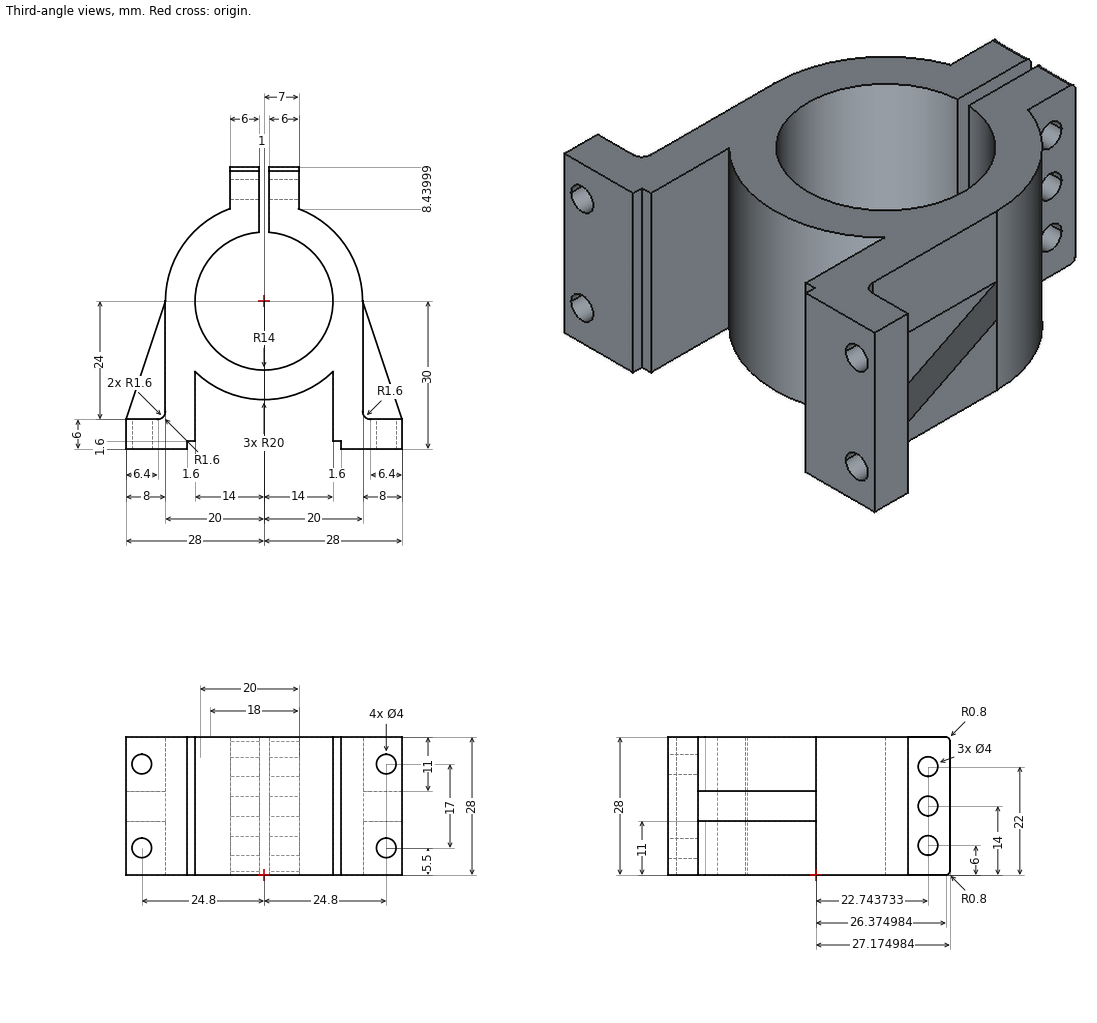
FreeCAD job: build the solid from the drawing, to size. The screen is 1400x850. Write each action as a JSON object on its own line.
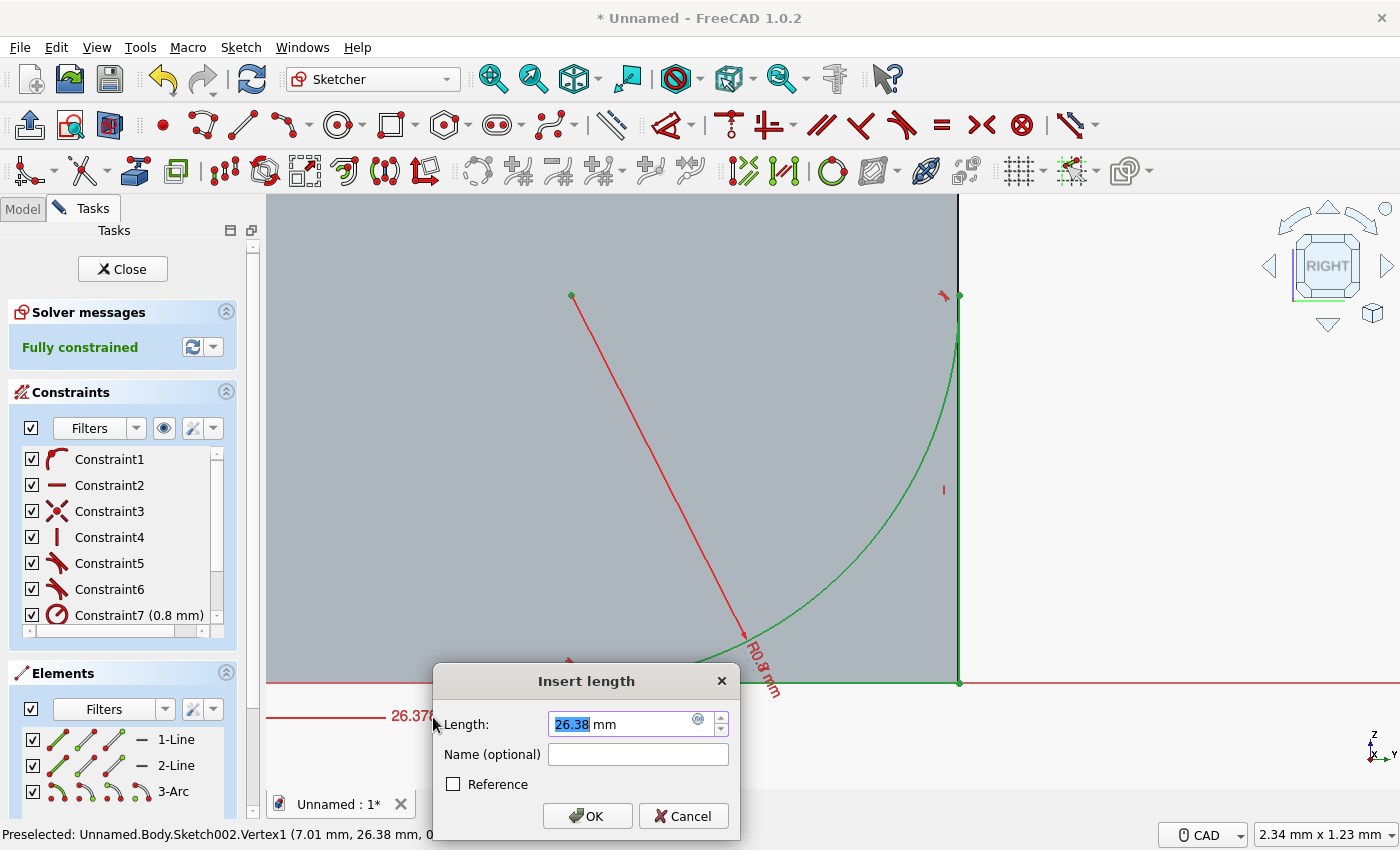
{"action": "type", "text": "26.374984"}
{"action": "key", "text": "Return"}
{"action": "key", "text": "Escape"}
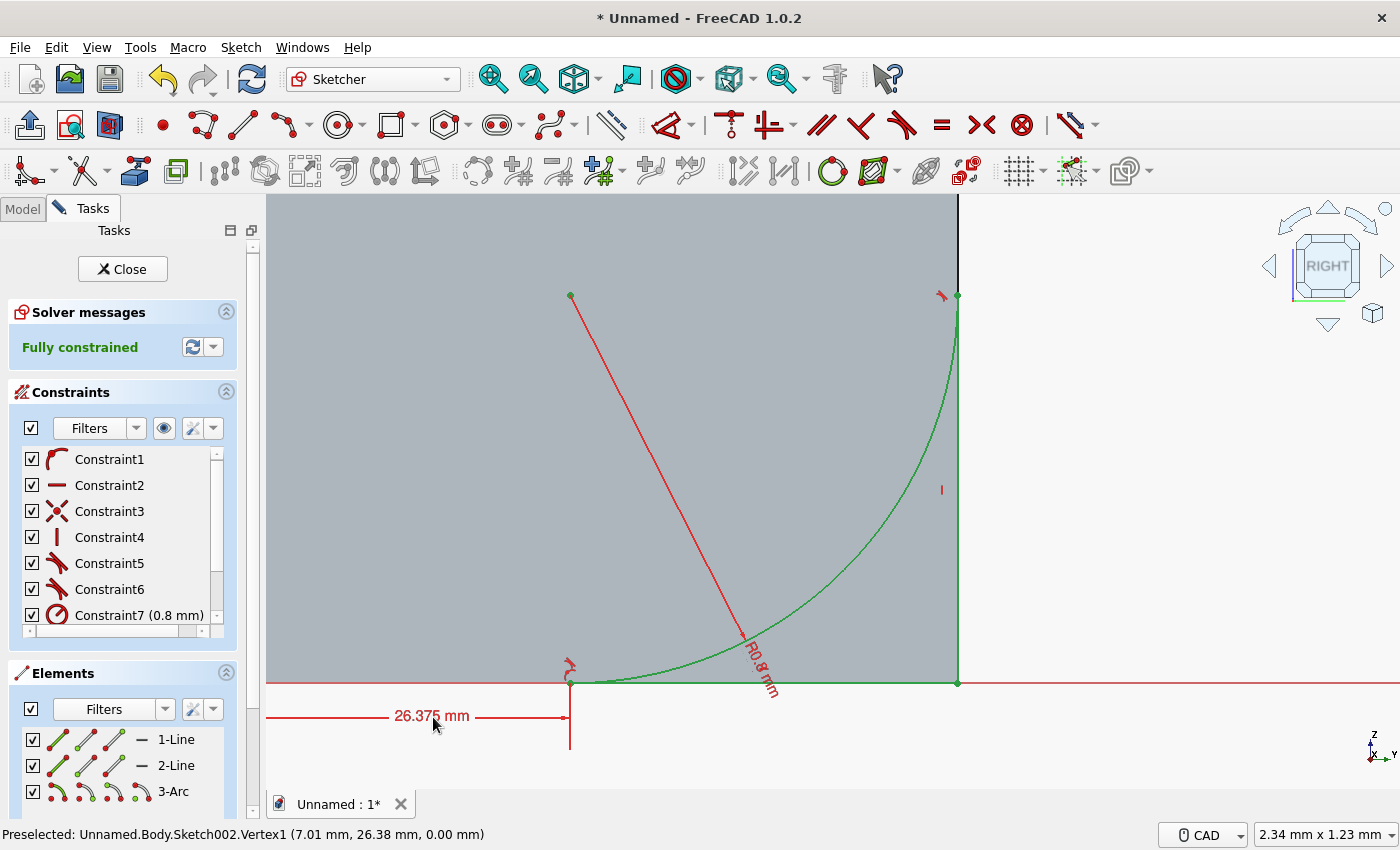
{"action": "left_click", "coordinate": [123, 269]}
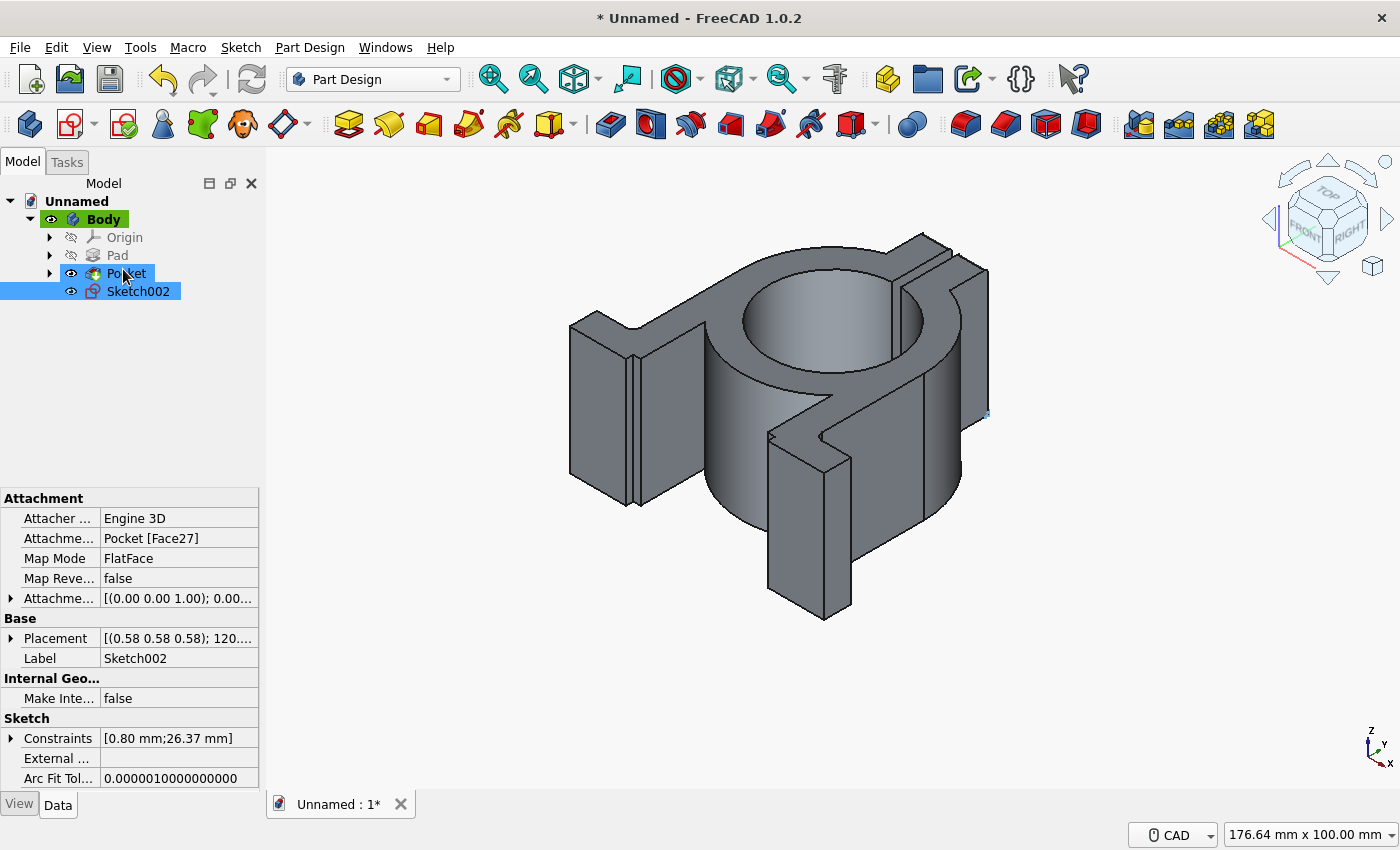
{"action": "left_click", "coordinate": [612, 124]}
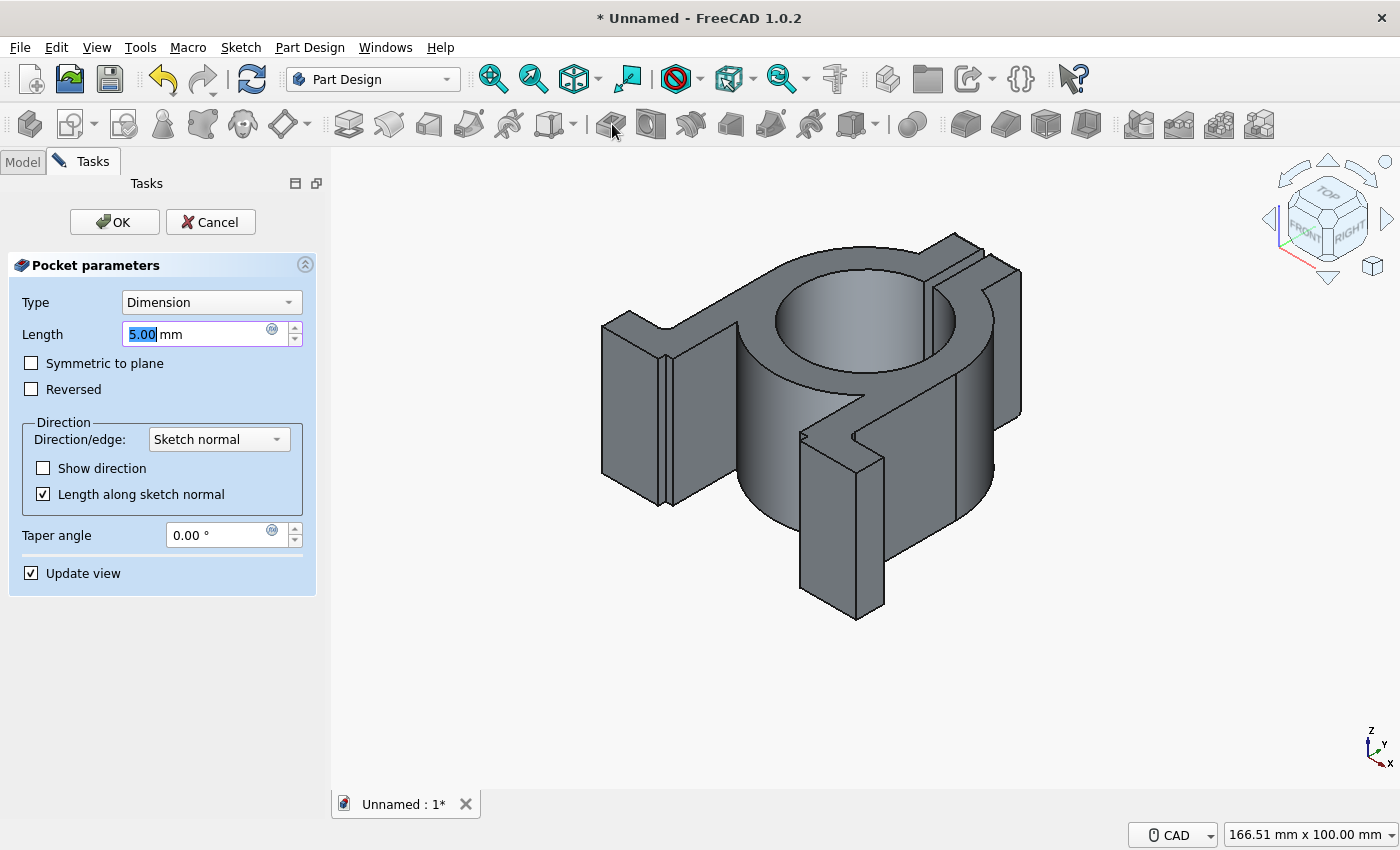
{"action": "type", "text": "18"}
{"action": "key", "text": "Tab"}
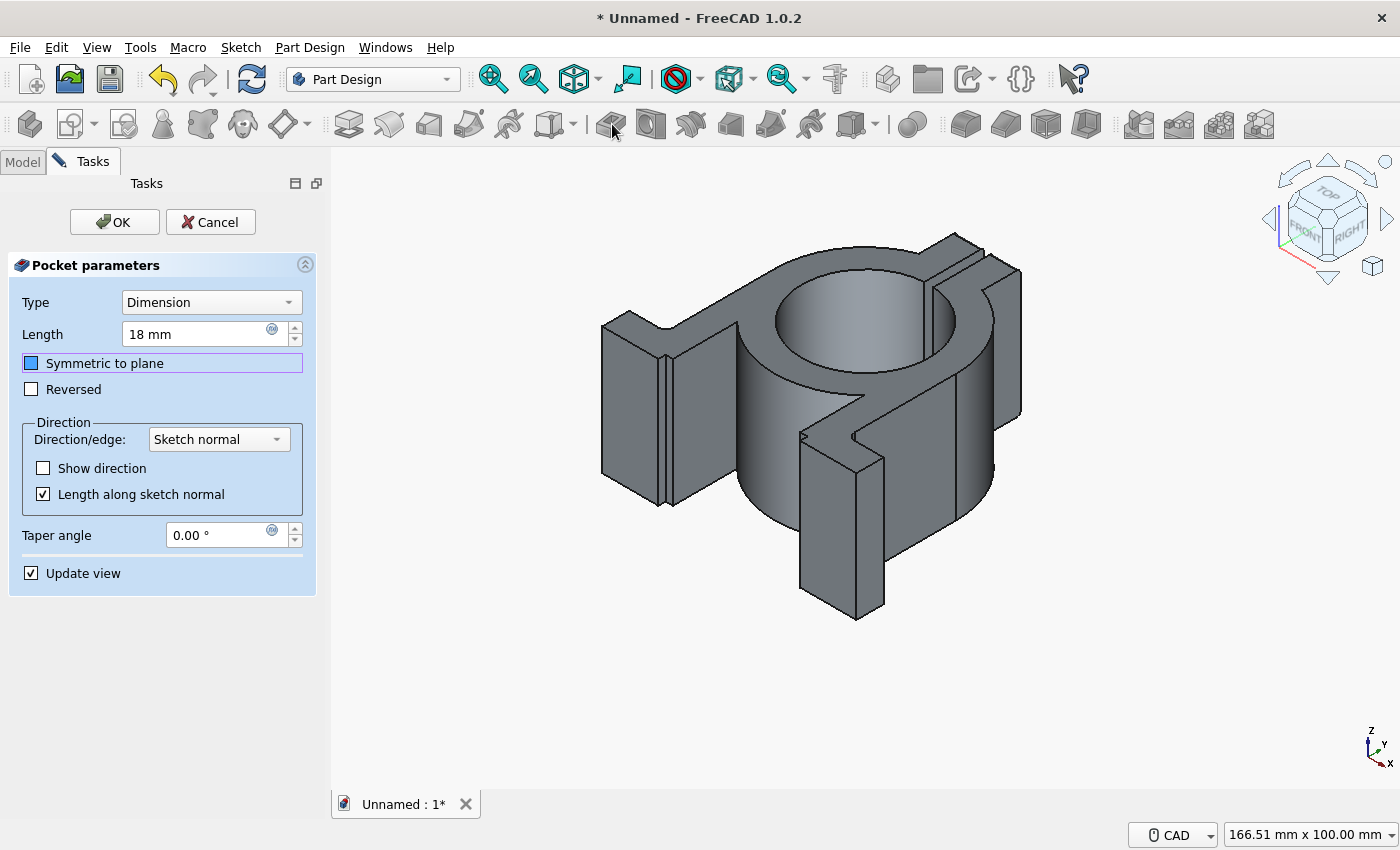
{"action": "left_click", "coordinate": [115, 222]}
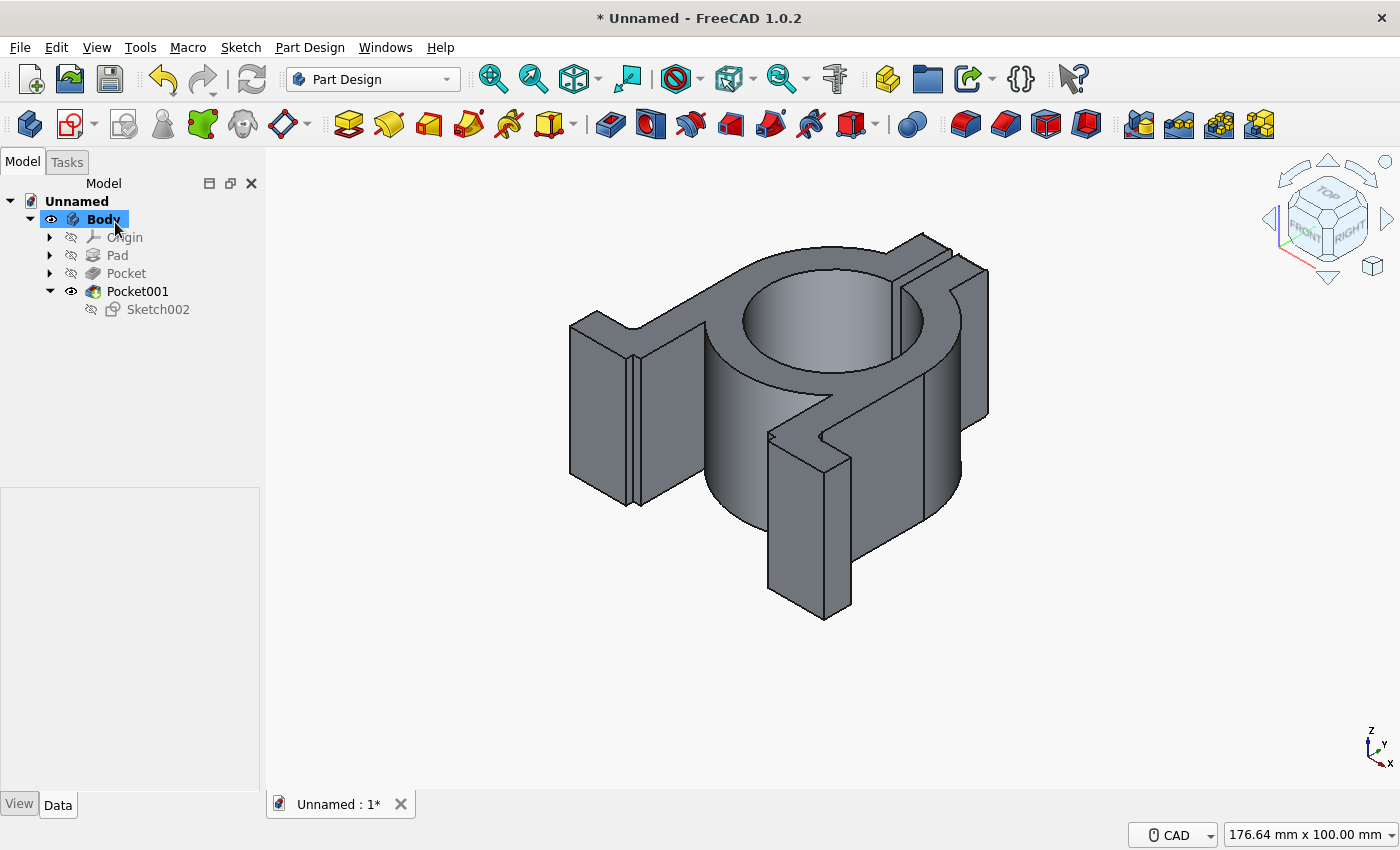
{"action": "key", "text": "5"}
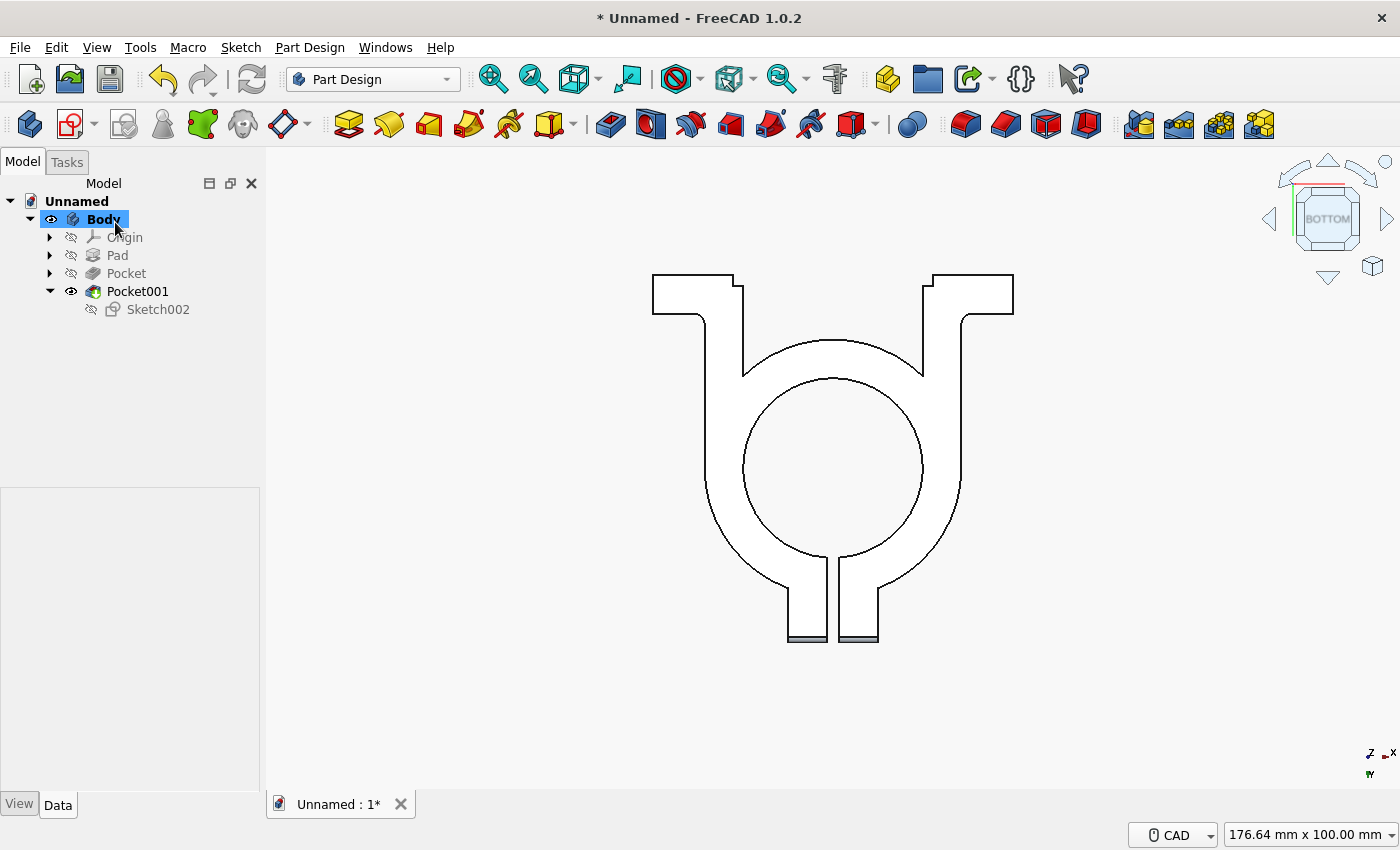
{"action": "left_click", "coordinate": [936, 404]}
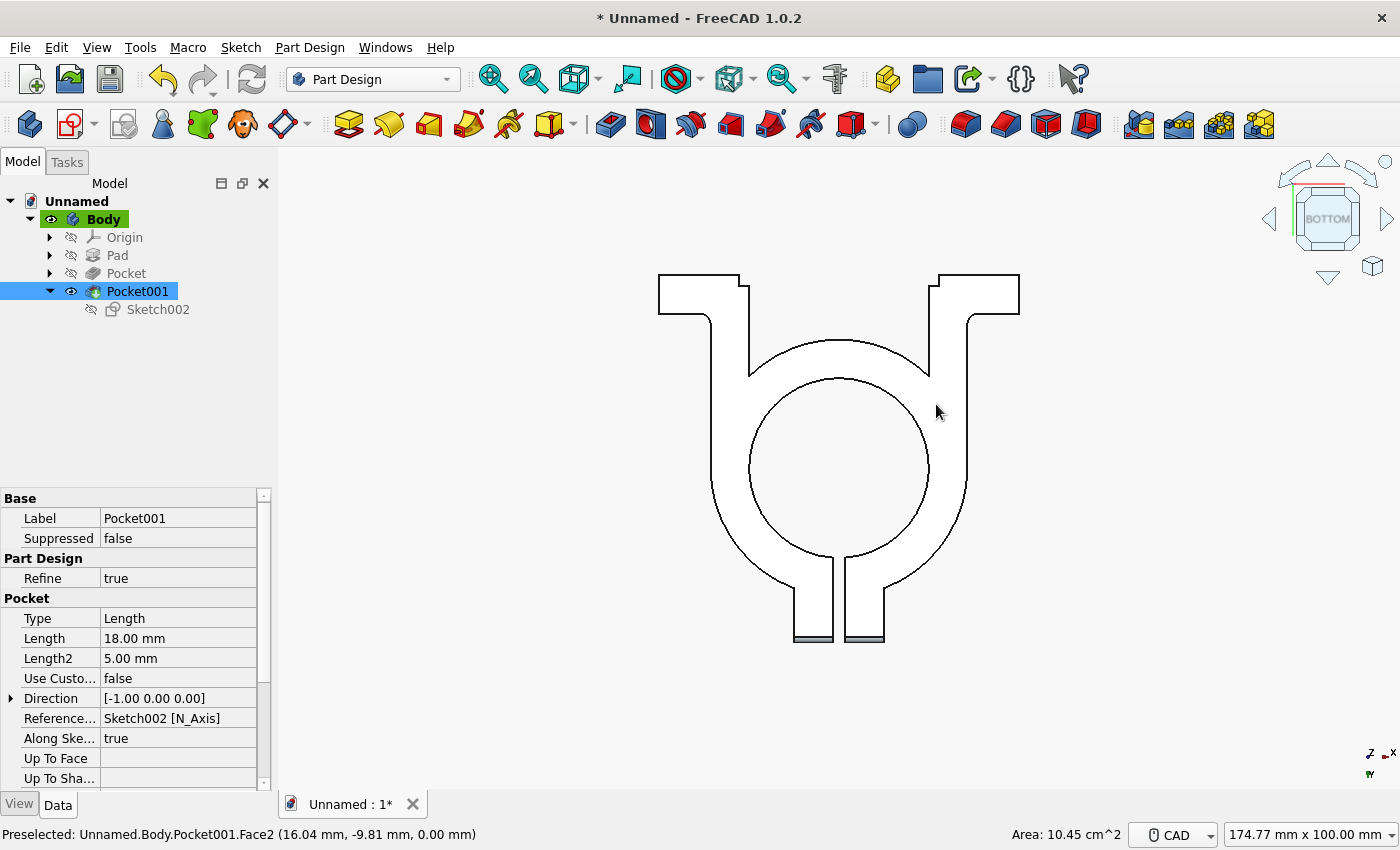
{"action": "left_click", "coordinate": [70, 124]}